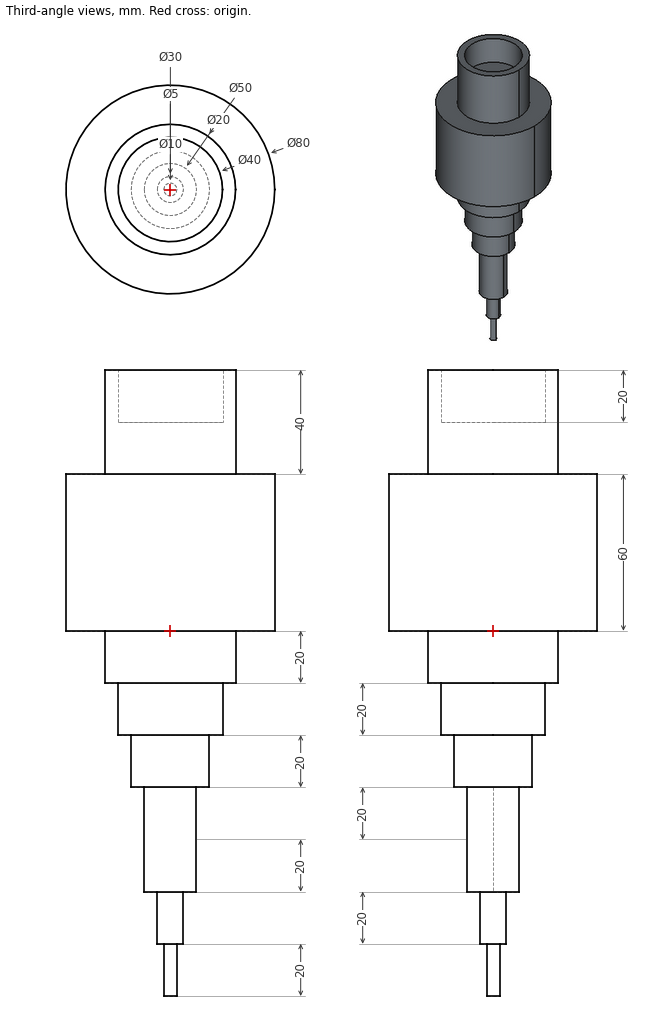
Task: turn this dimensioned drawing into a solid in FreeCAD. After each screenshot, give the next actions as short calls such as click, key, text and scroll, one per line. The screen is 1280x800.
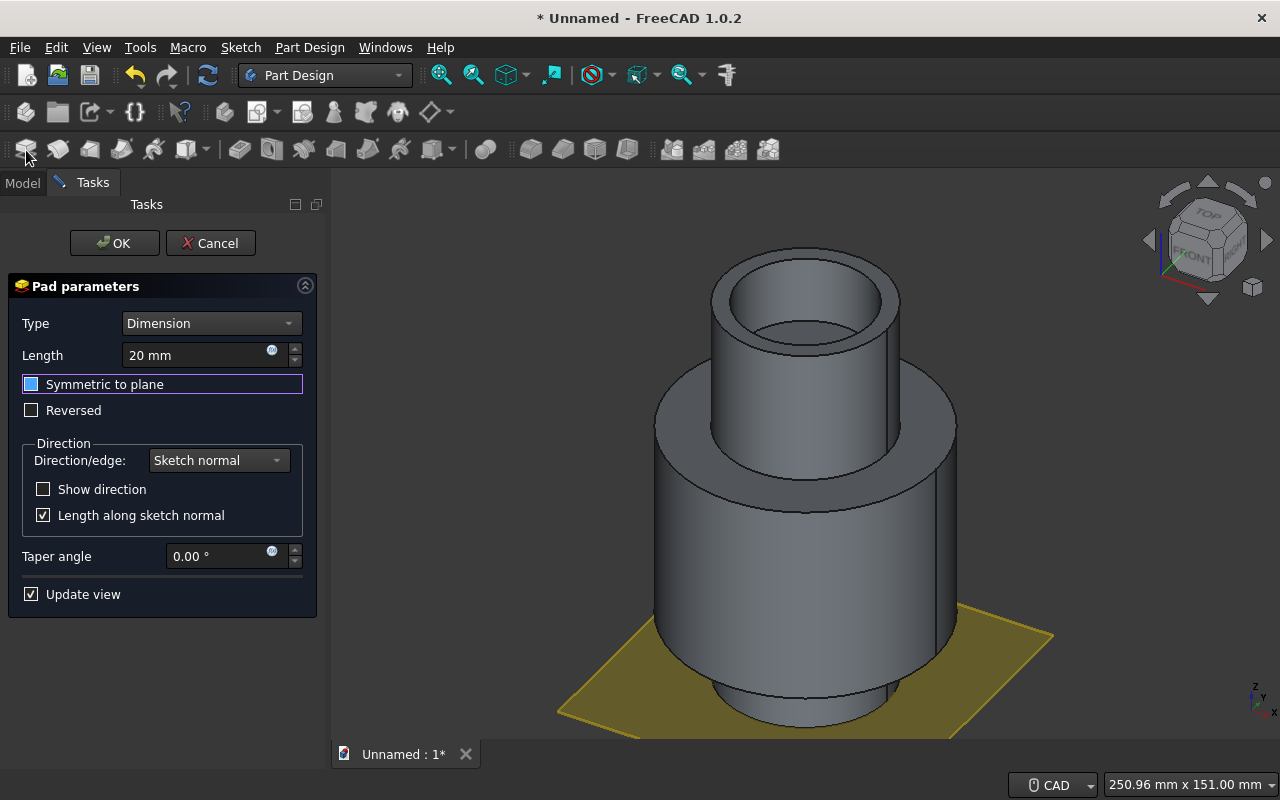
click(115, 243)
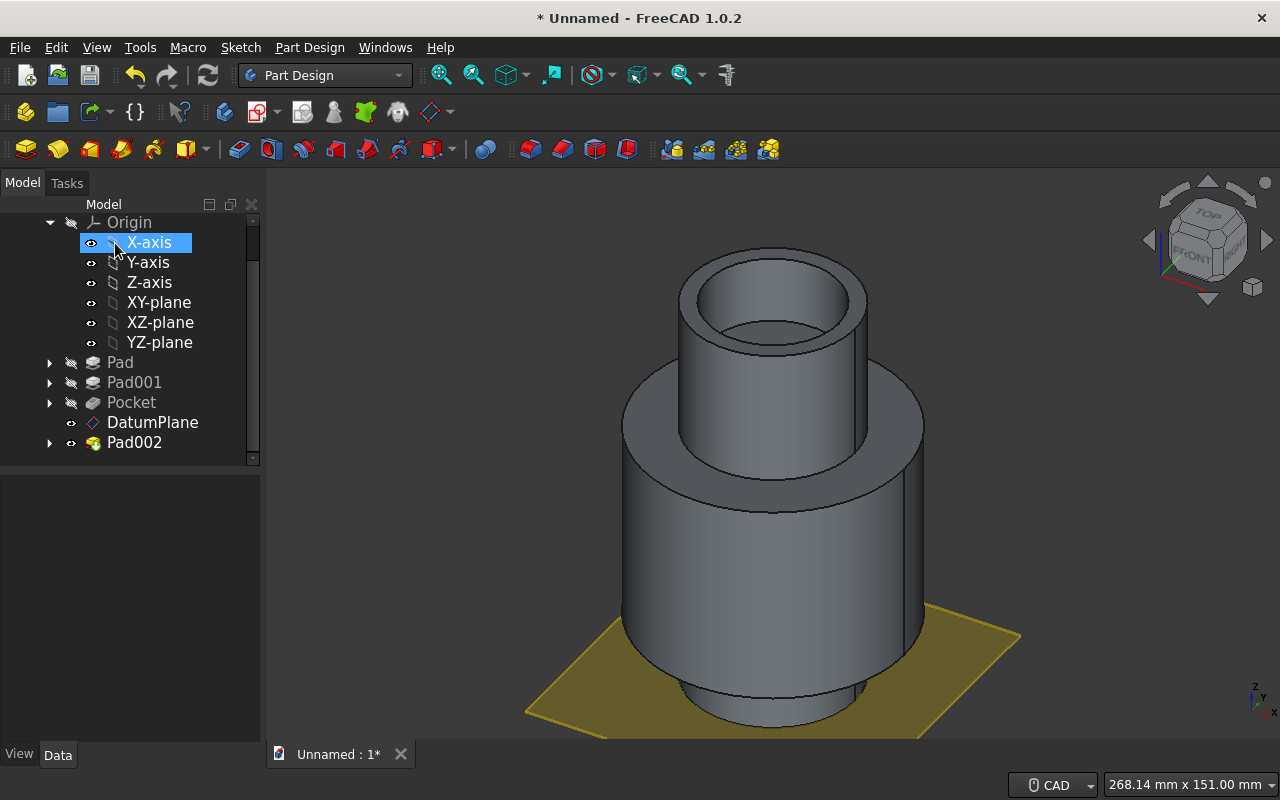
click(116, 423)
key(space)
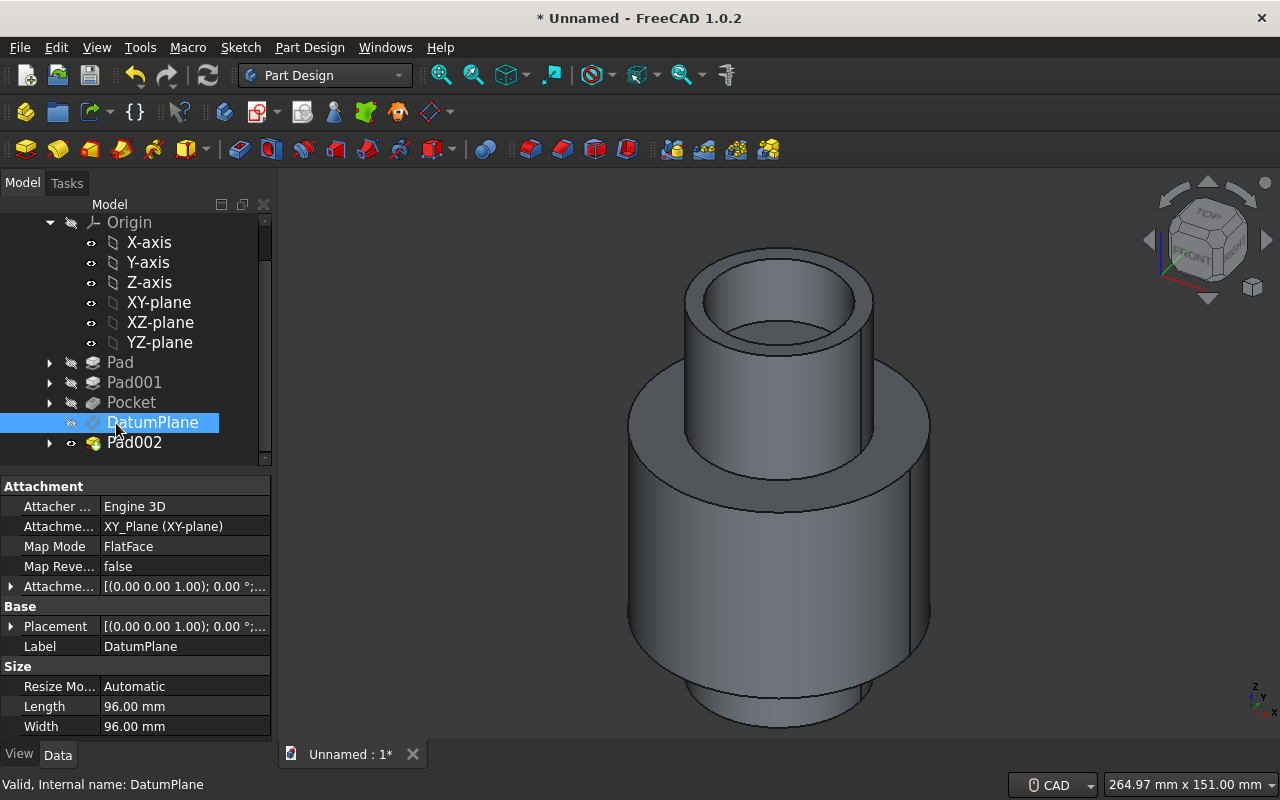
click(442, 76)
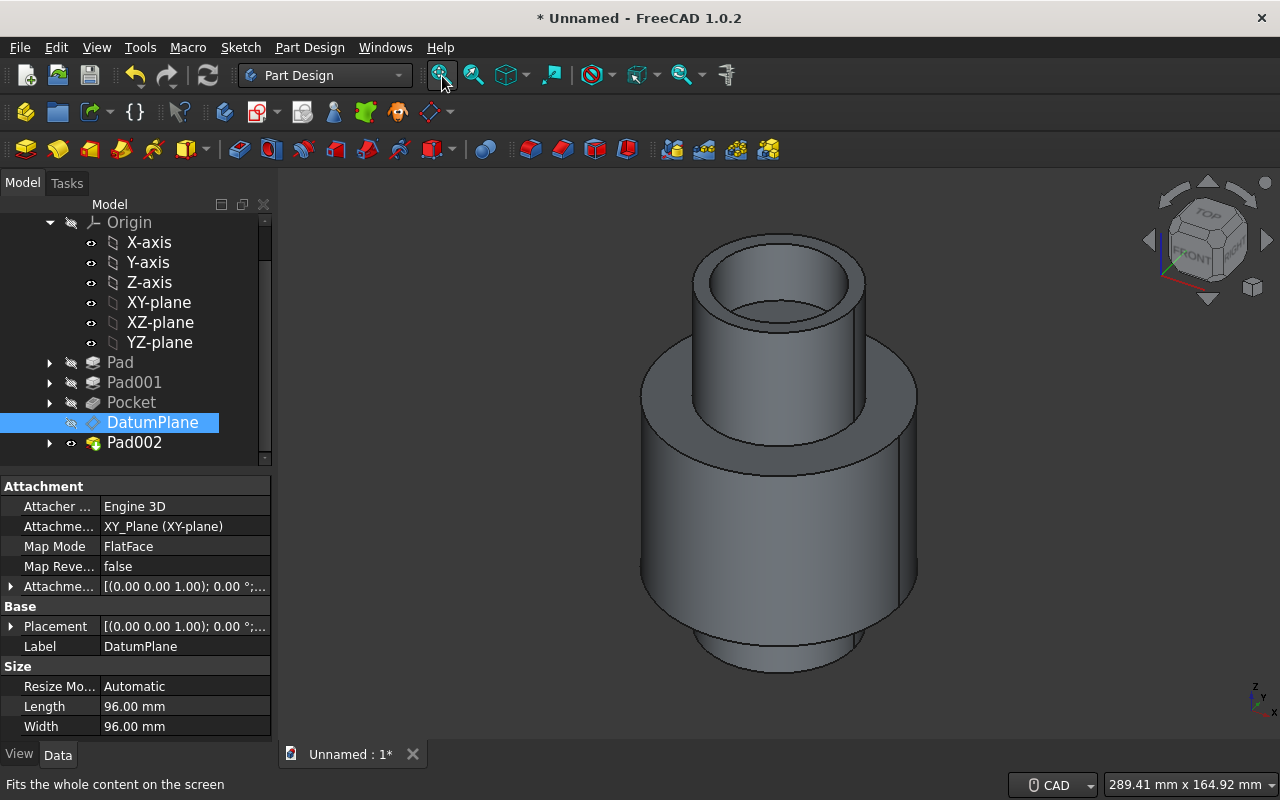
key(5)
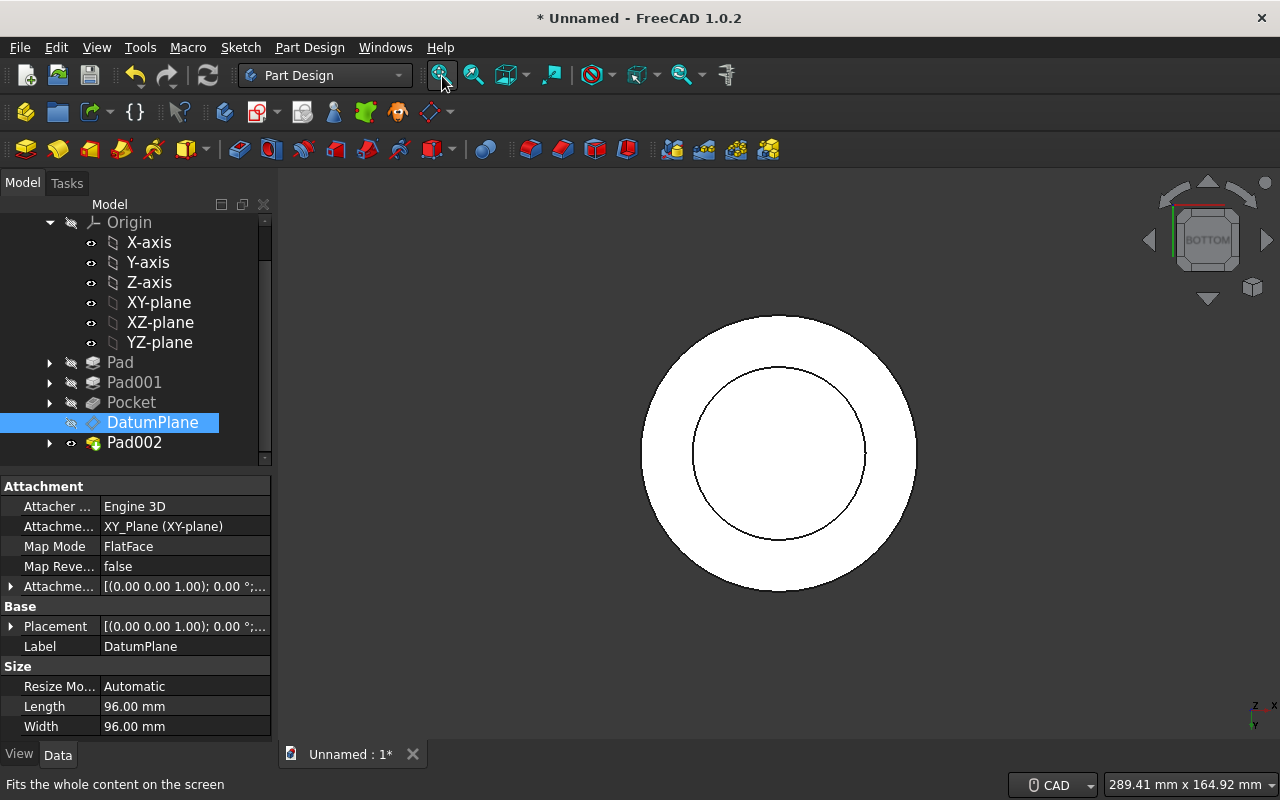
click(779, 452)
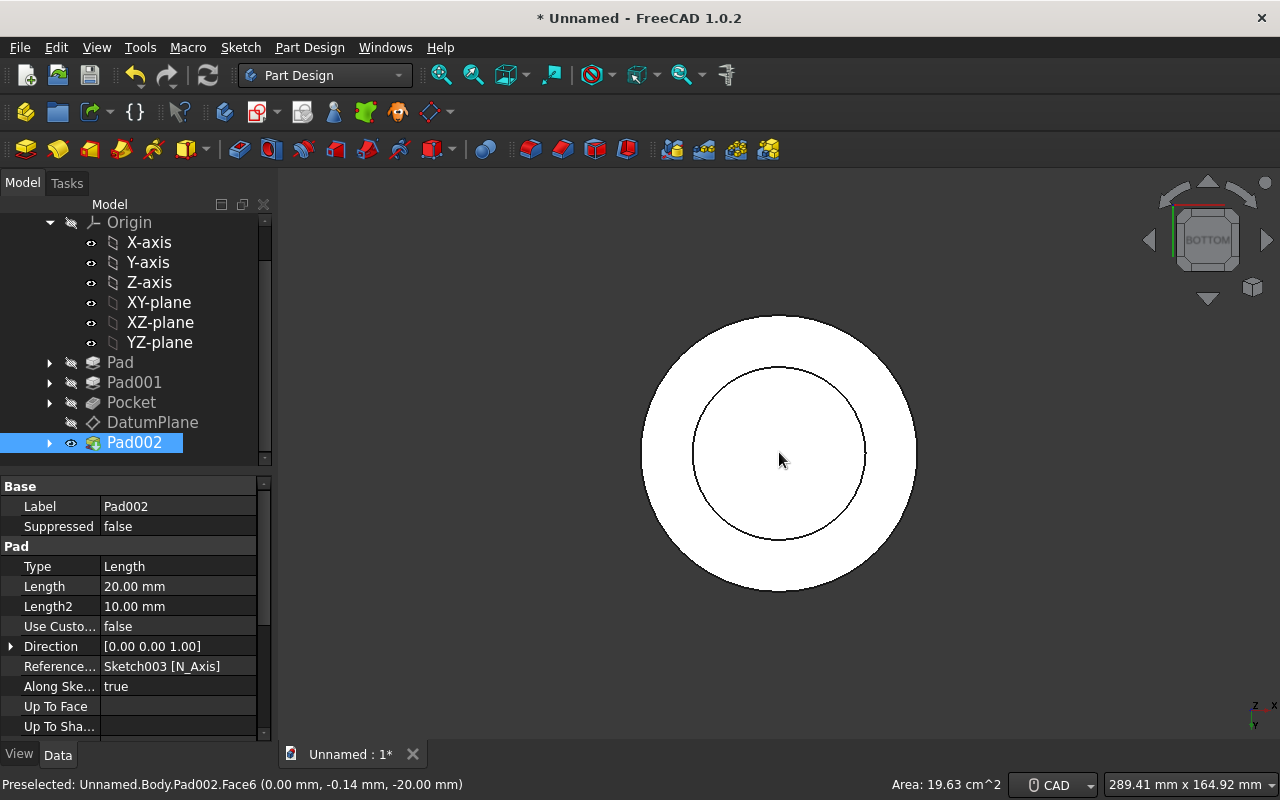
click(258, 112)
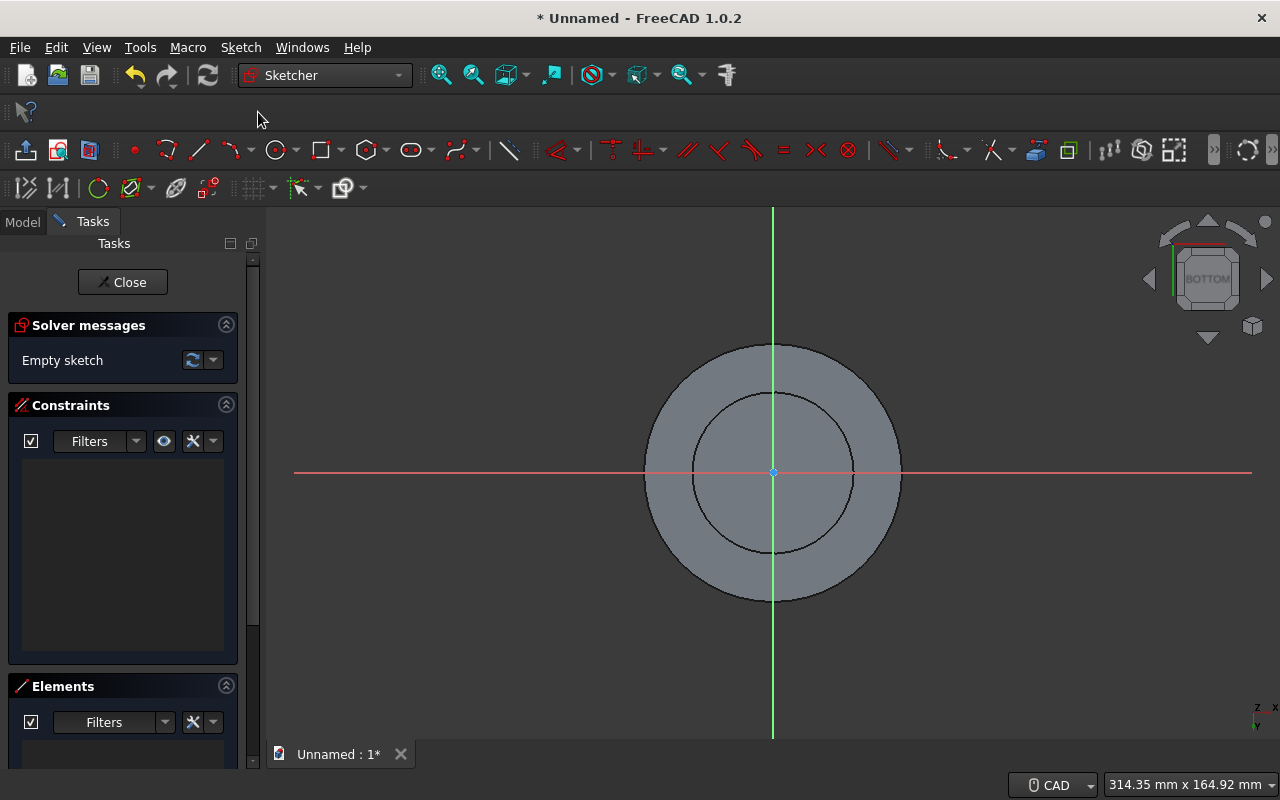
scroll(813, 473, up, 5)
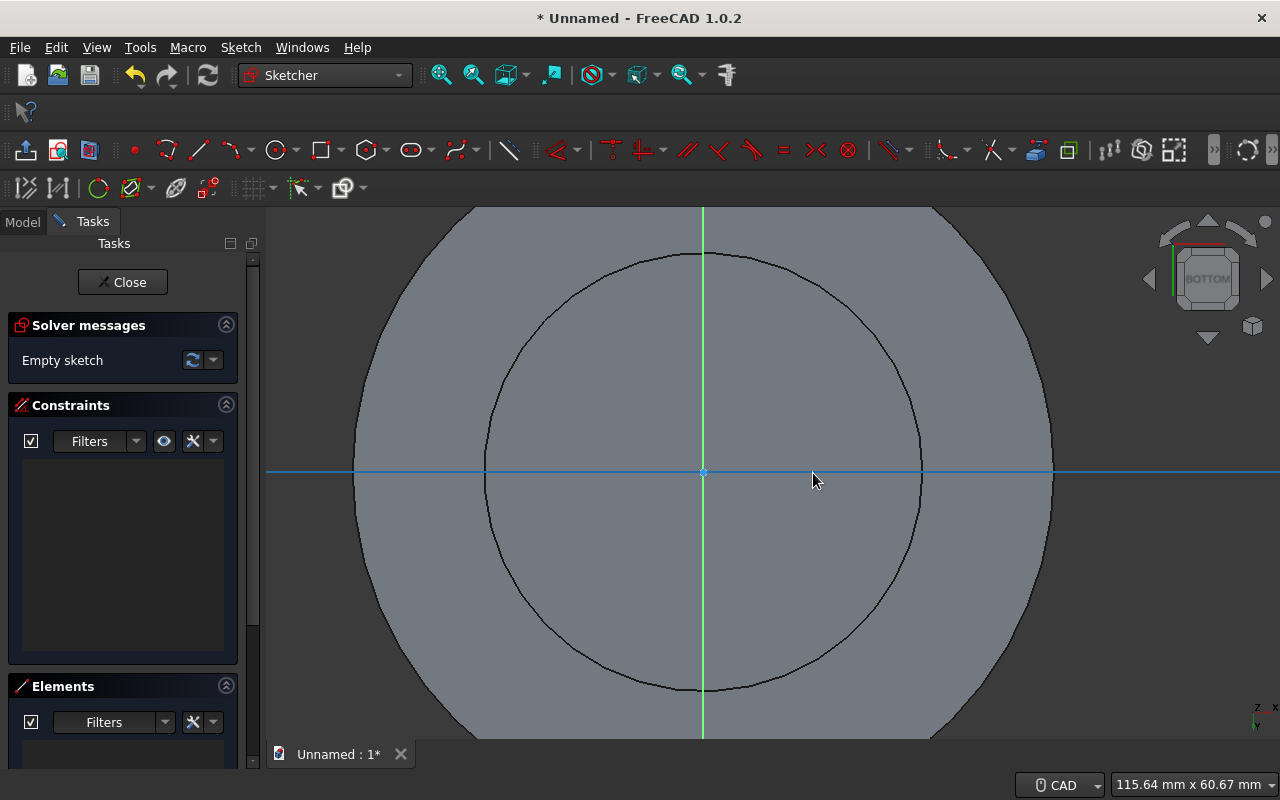
click(276, 150)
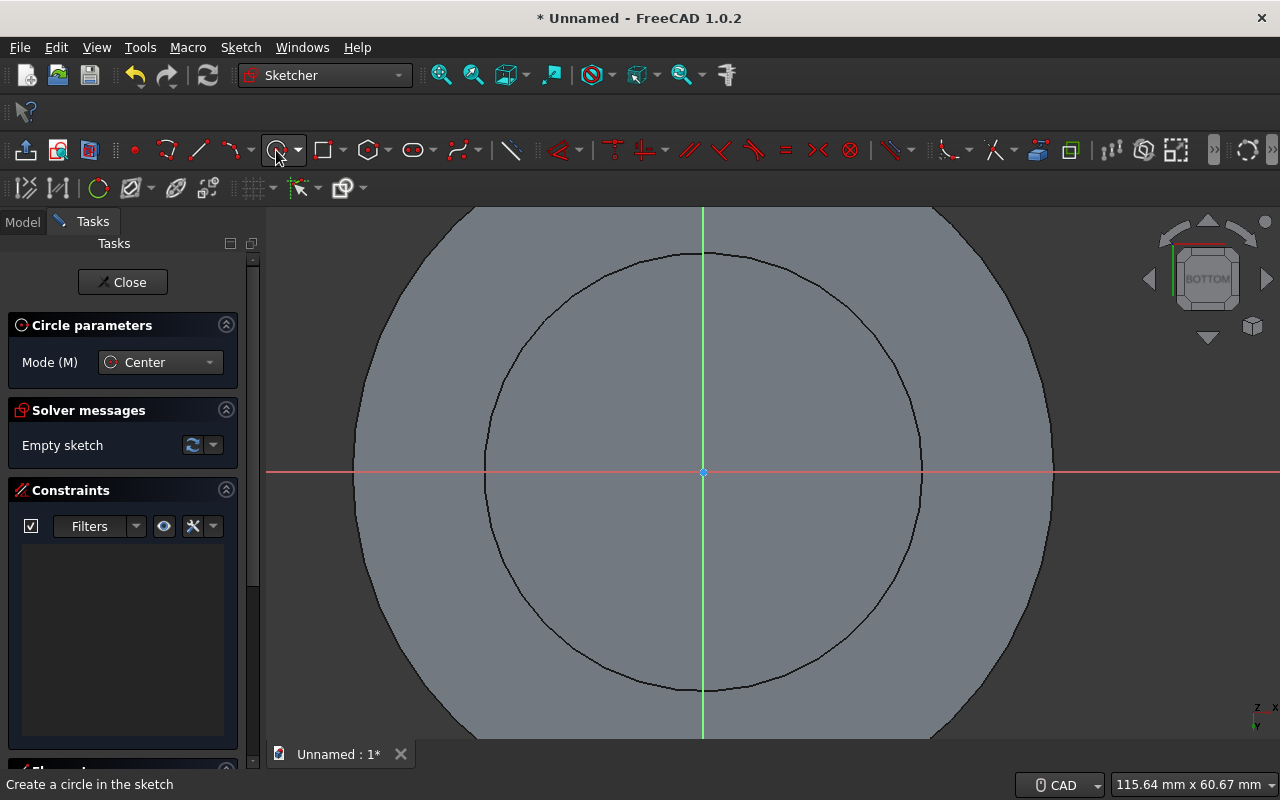
click(703, 472)
click(827, 348)
key(Escape)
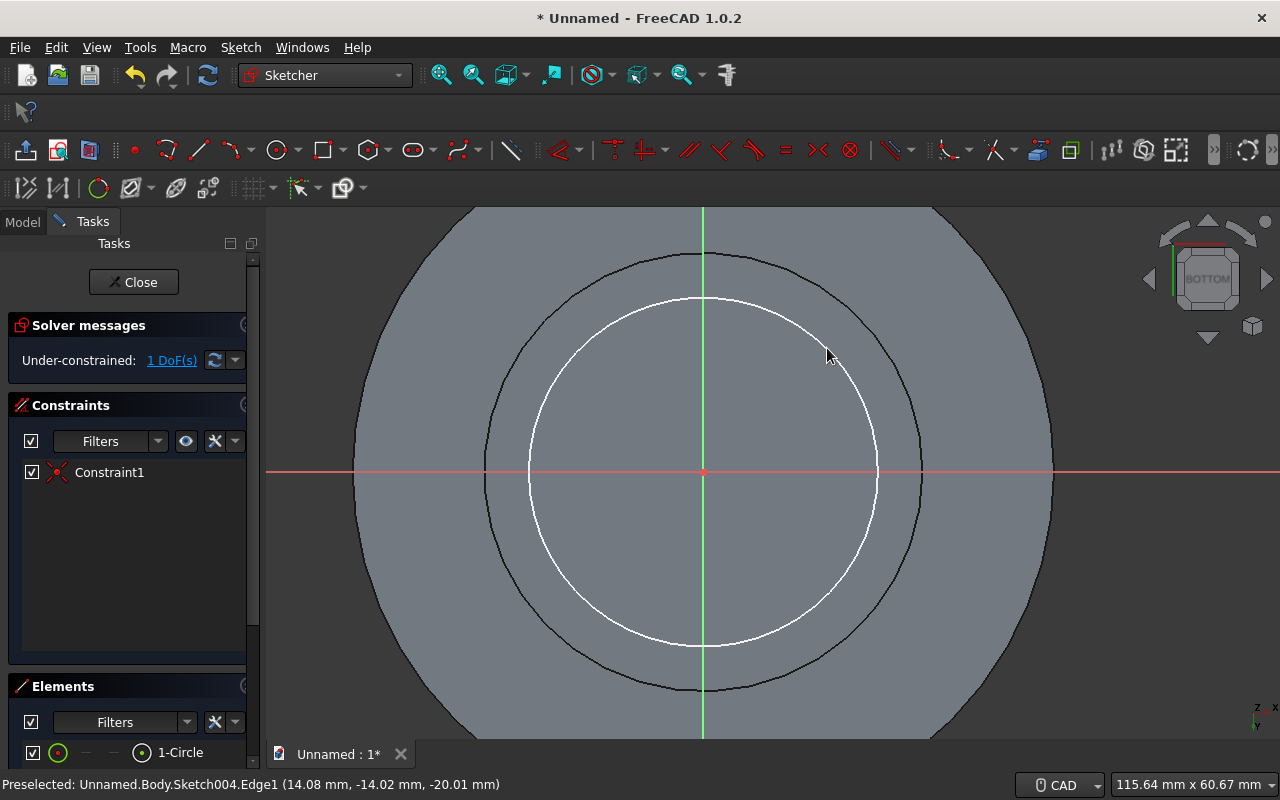
click(558, 150)